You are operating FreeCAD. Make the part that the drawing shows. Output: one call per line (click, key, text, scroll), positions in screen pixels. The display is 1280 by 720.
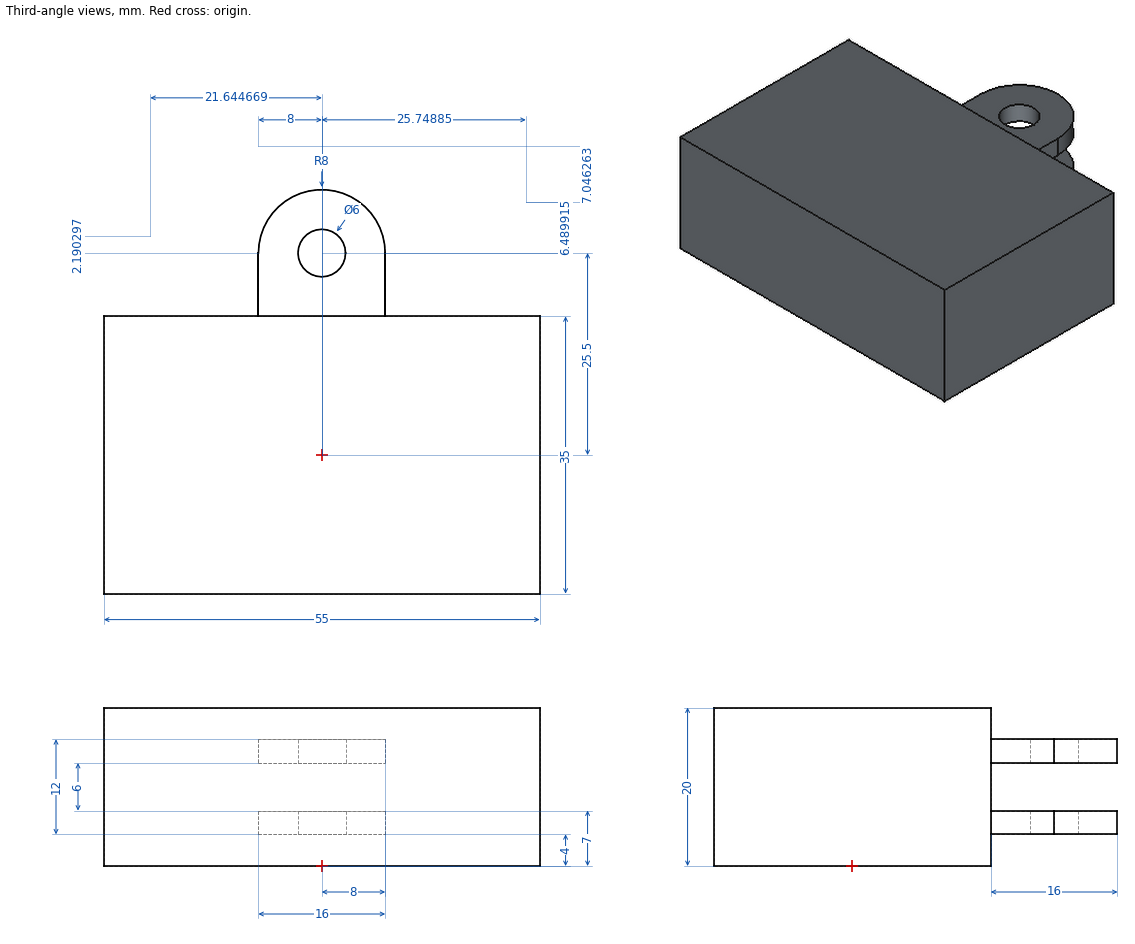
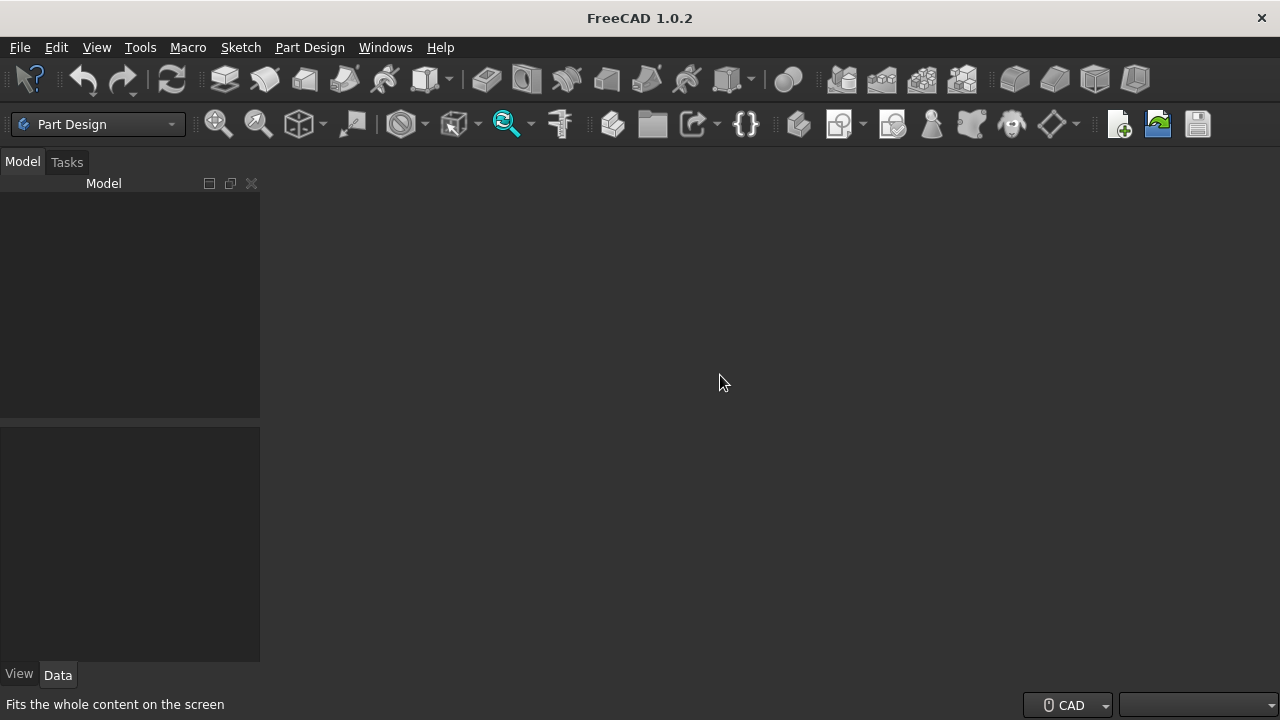
key(ctrl+n)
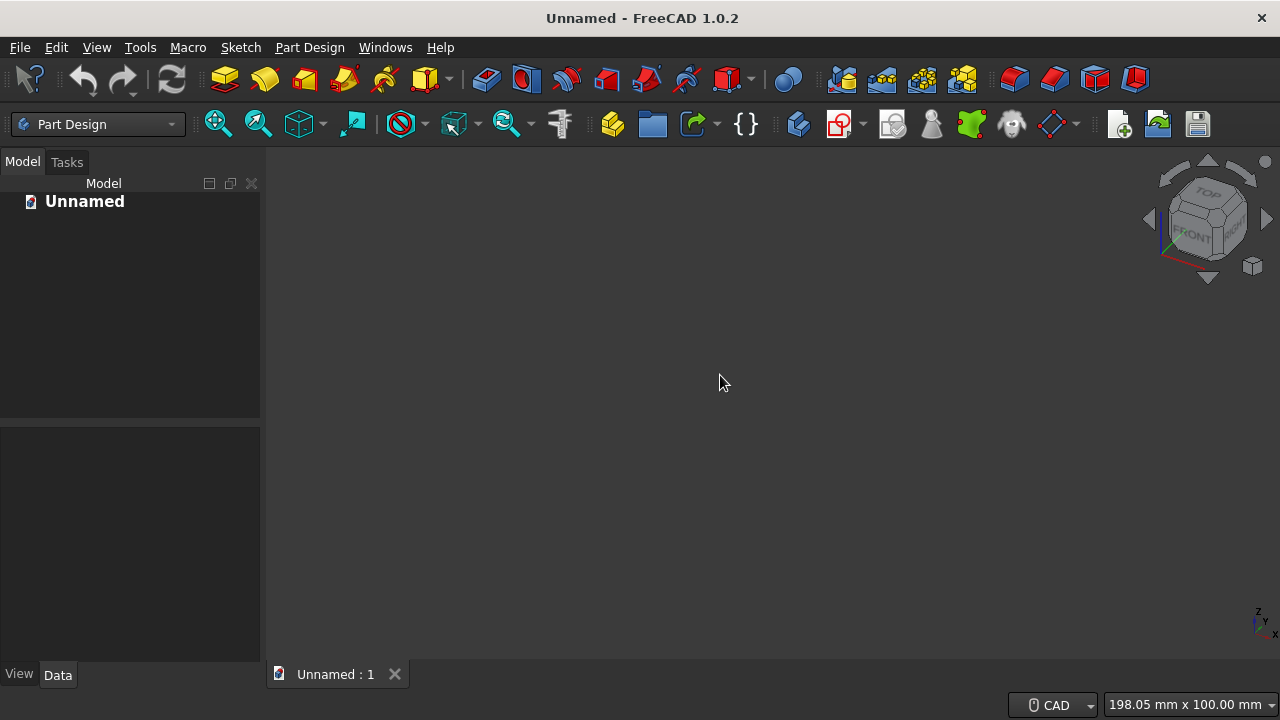
click(840, 124)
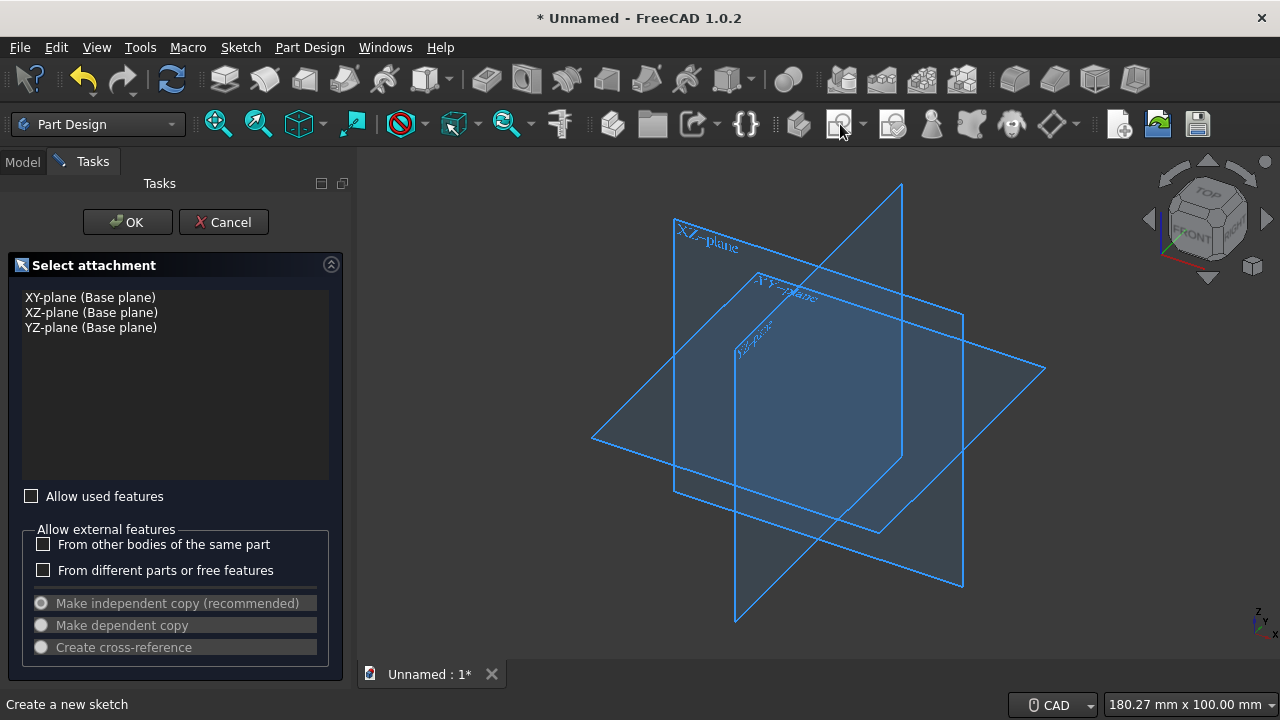
click(82, 298)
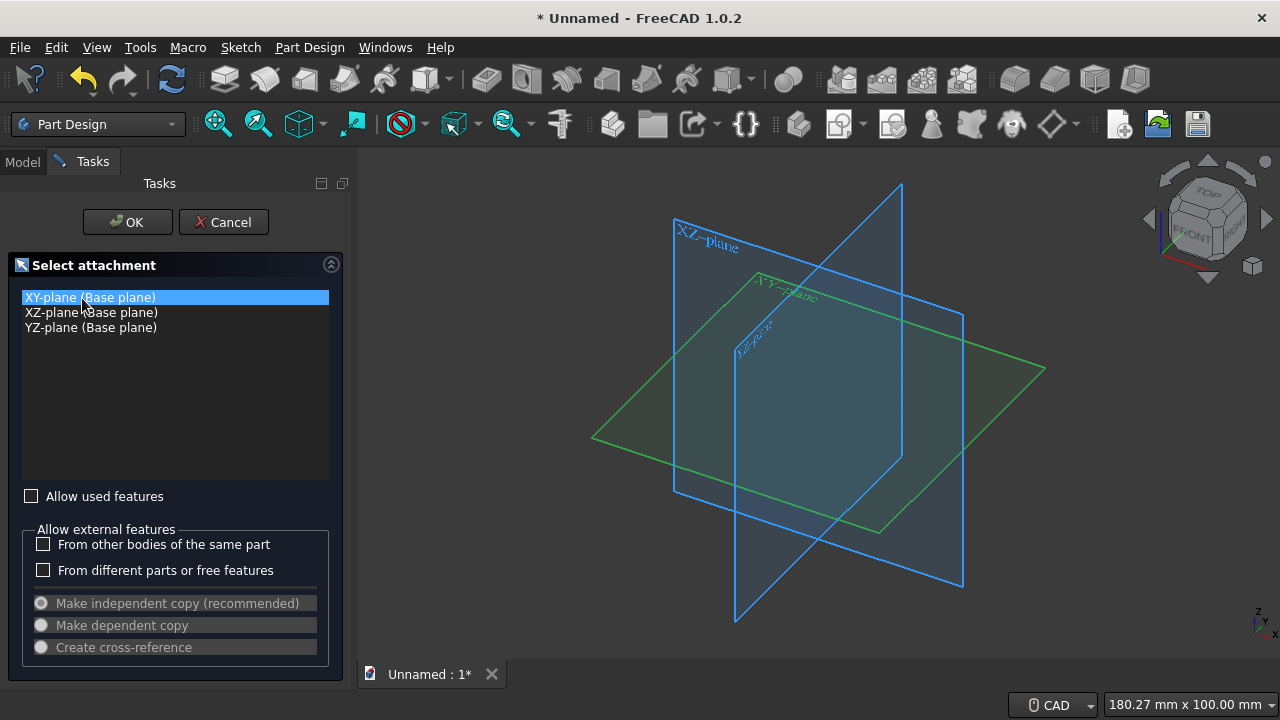
click(128, 222)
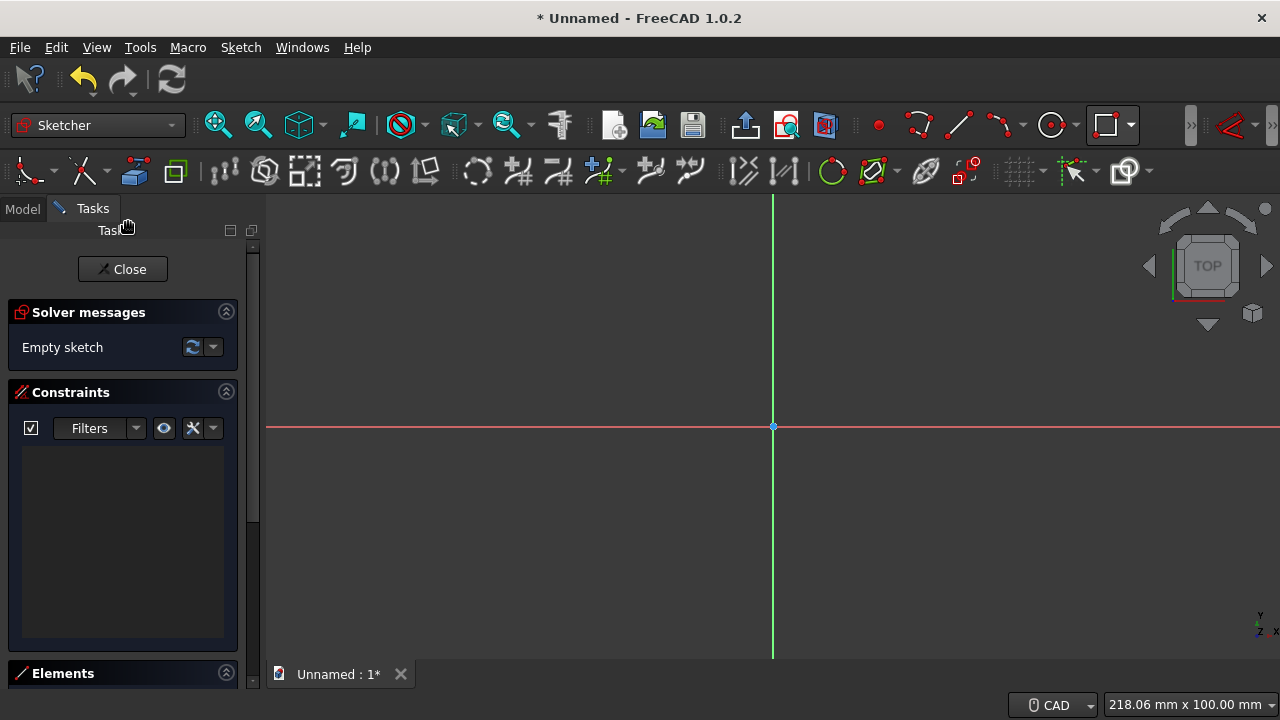
scroll(856, 426, up, 3)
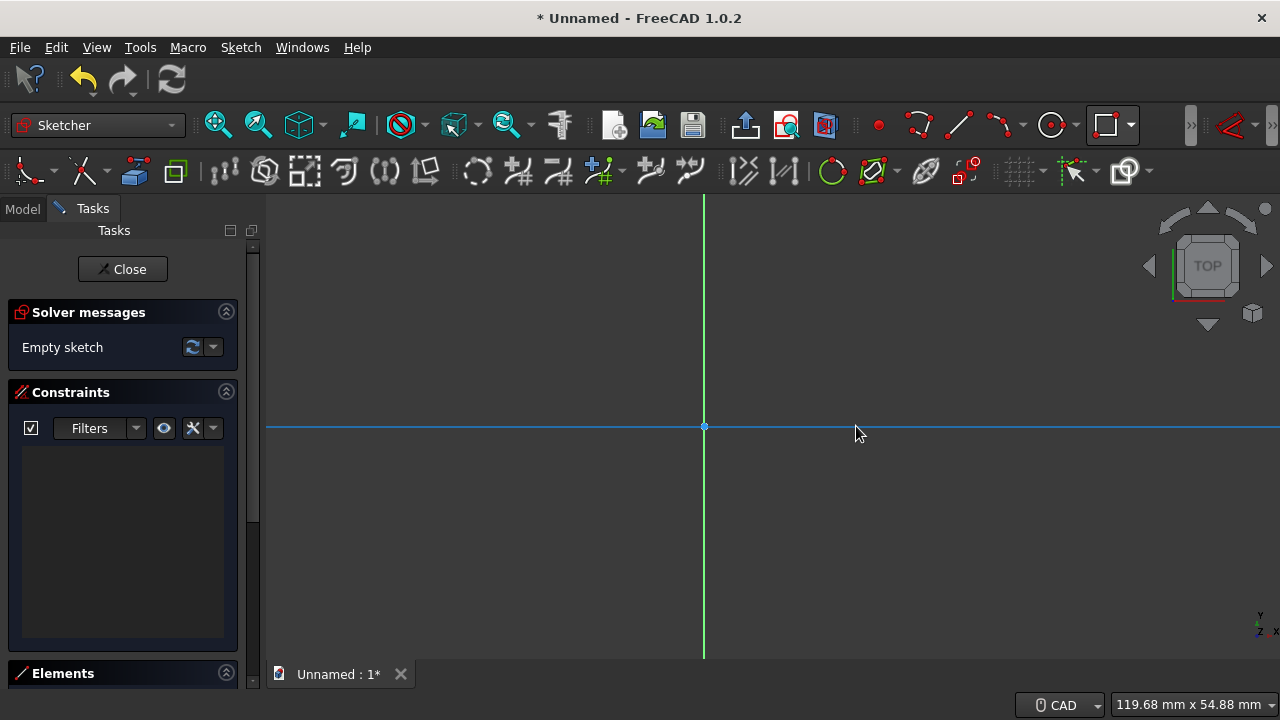
click(1134, 126)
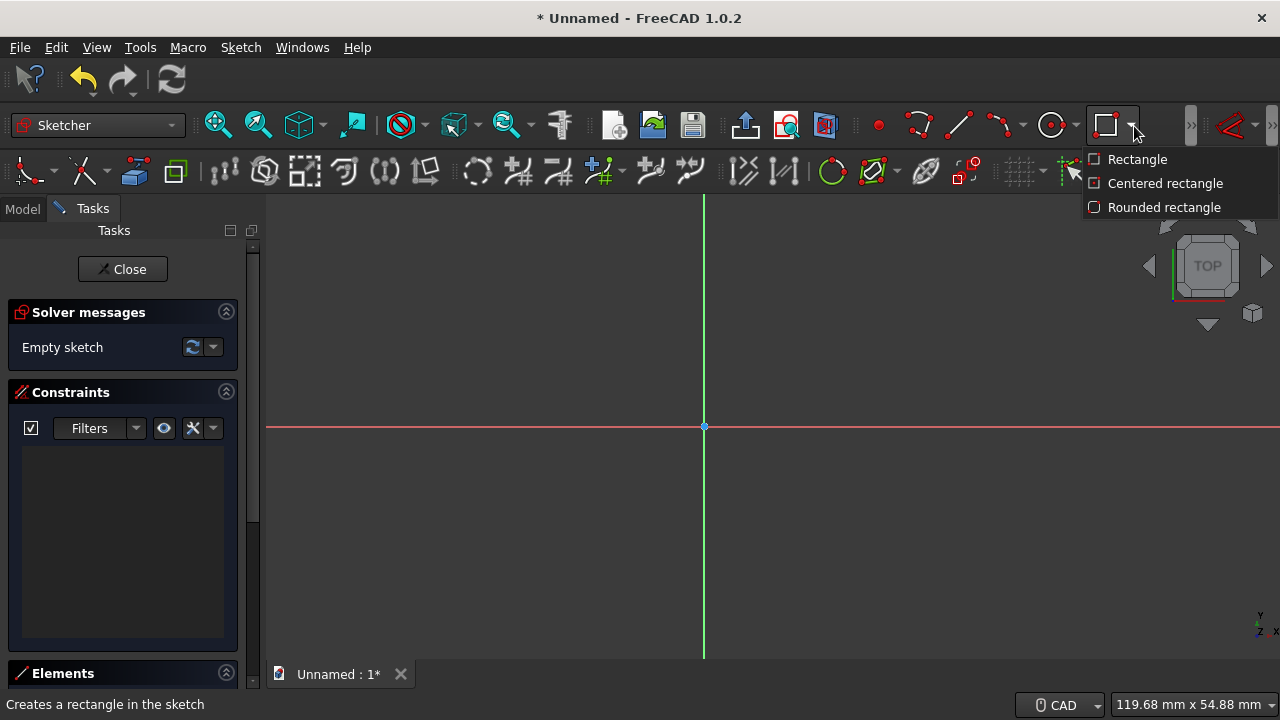
click(1180, 183)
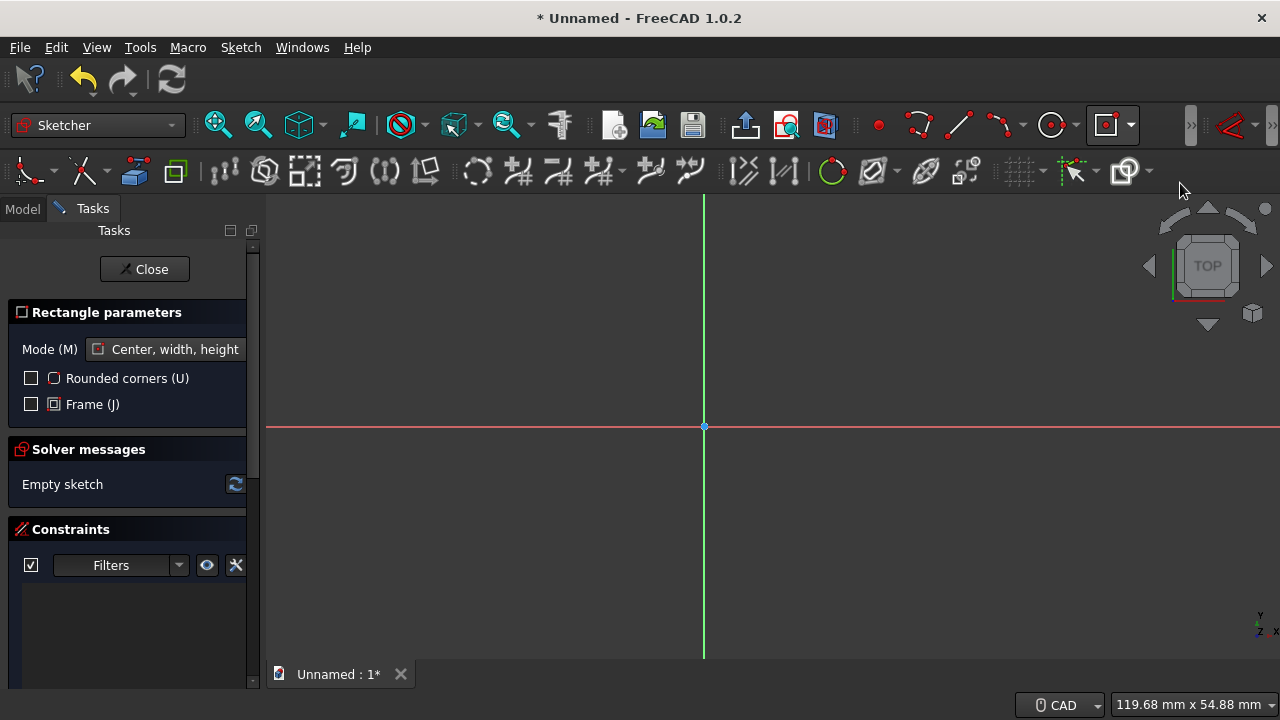
click(704, 426)
move(937, 278)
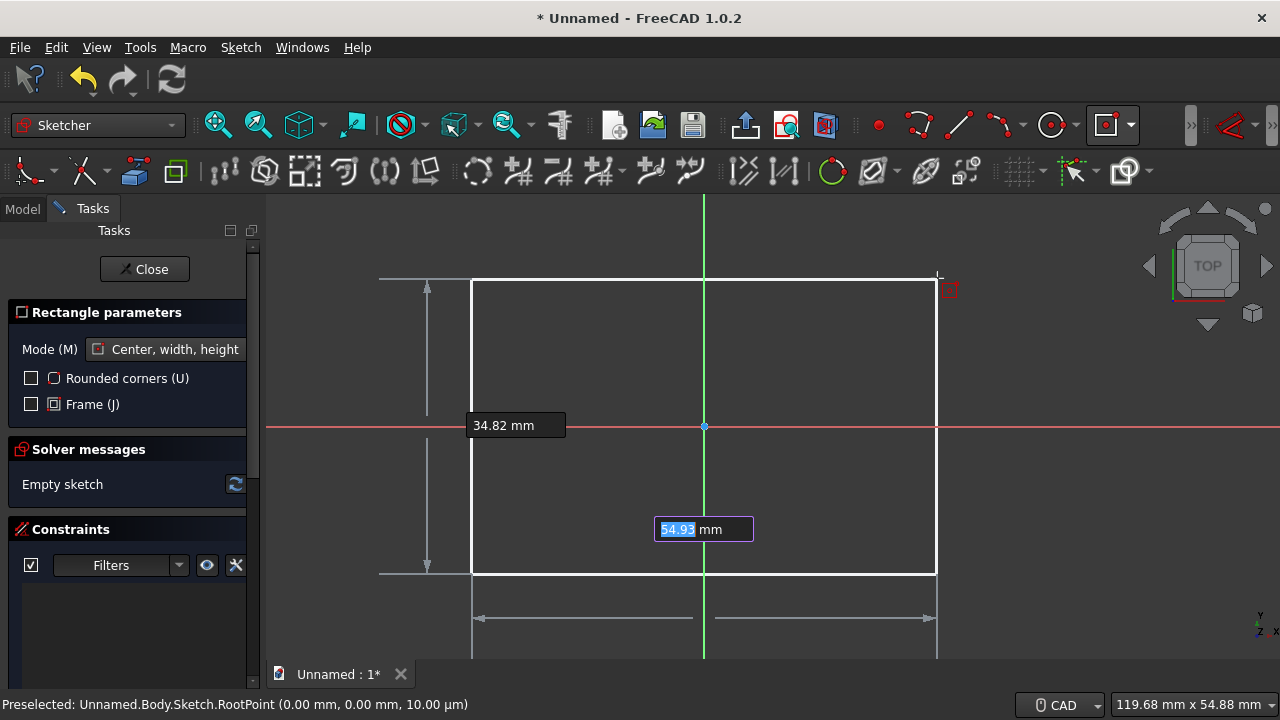
text(55)
key(Tab)
text(35)
key(Return)
key(Escape)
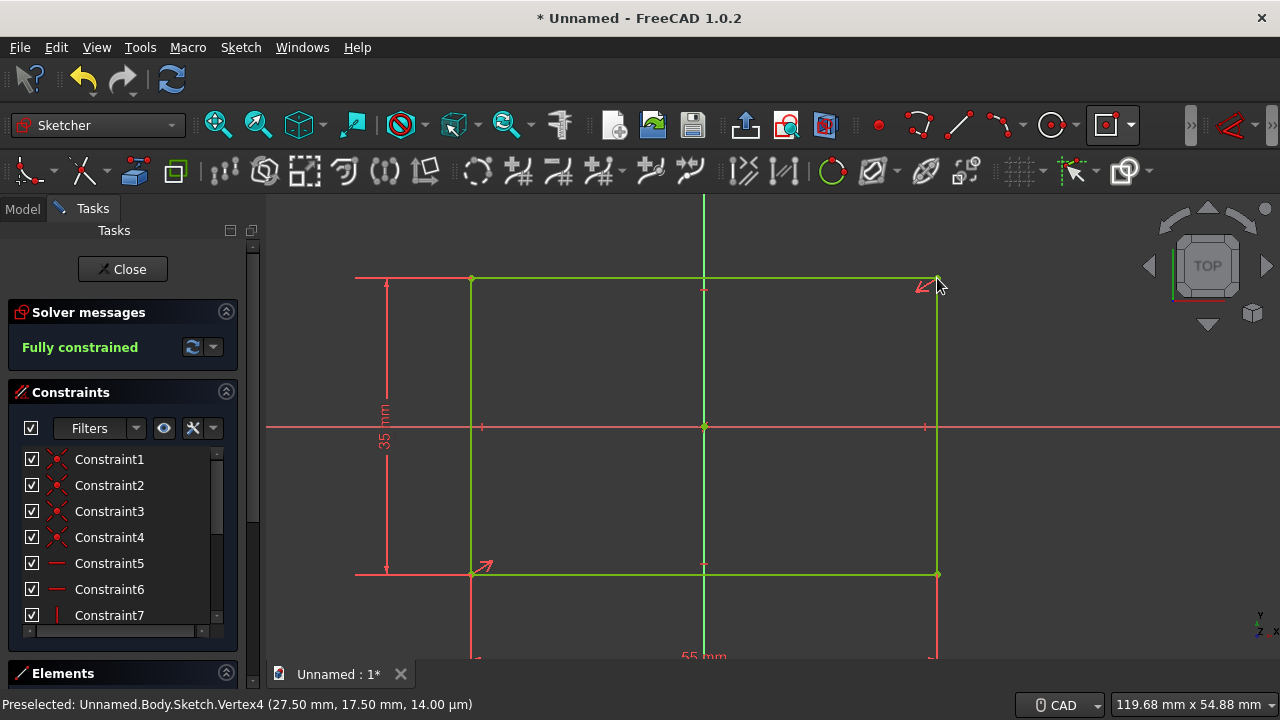
click(123, 269)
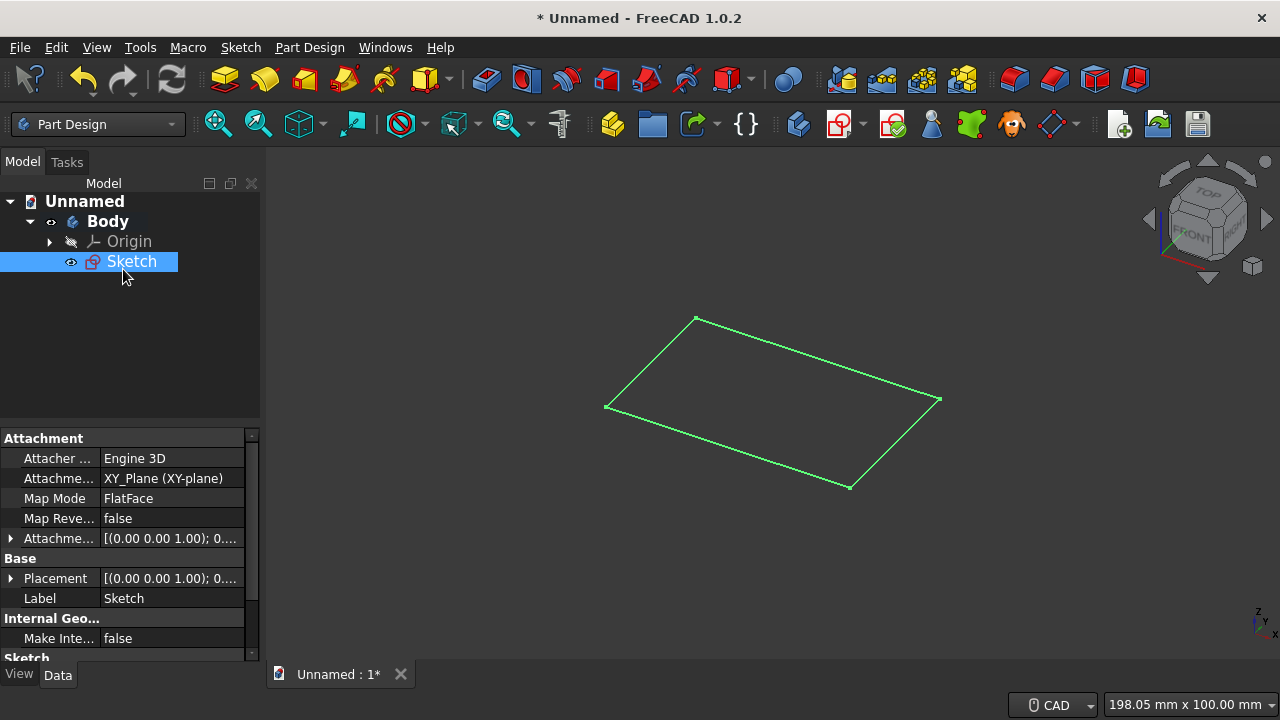
click(226, 80)